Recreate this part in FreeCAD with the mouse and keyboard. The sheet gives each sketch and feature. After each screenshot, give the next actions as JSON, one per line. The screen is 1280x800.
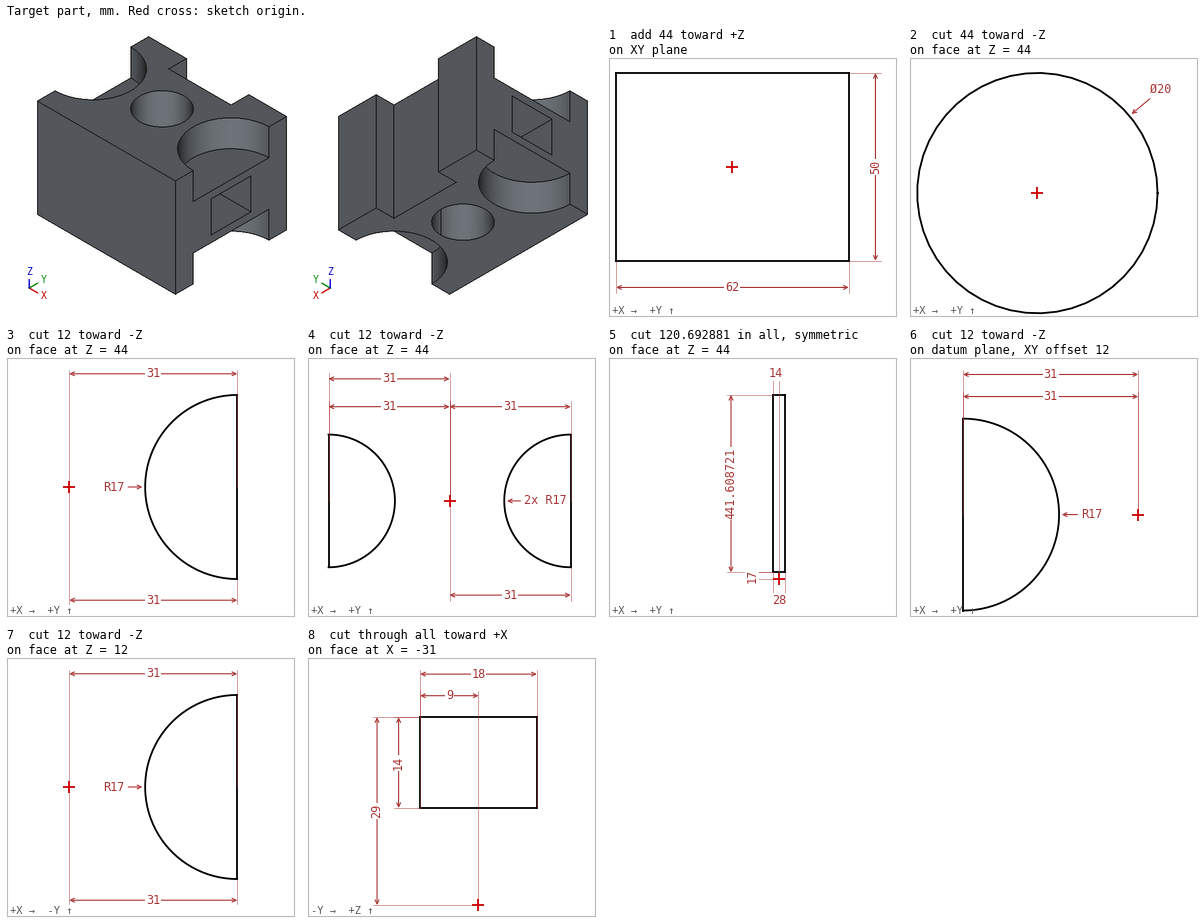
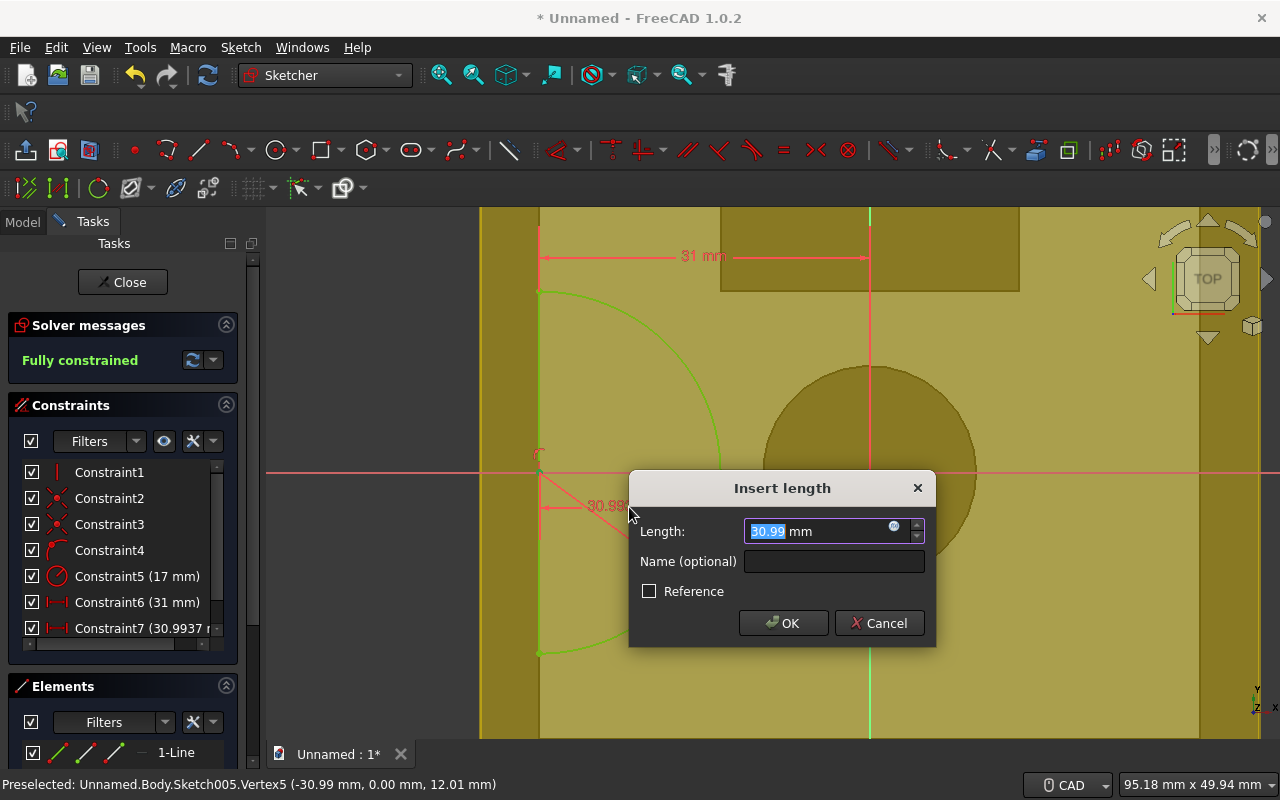
{"action": "type", "text": "31"}
{"action": "key", "text": "Return"}
{"action": "key", "text": "Escape"}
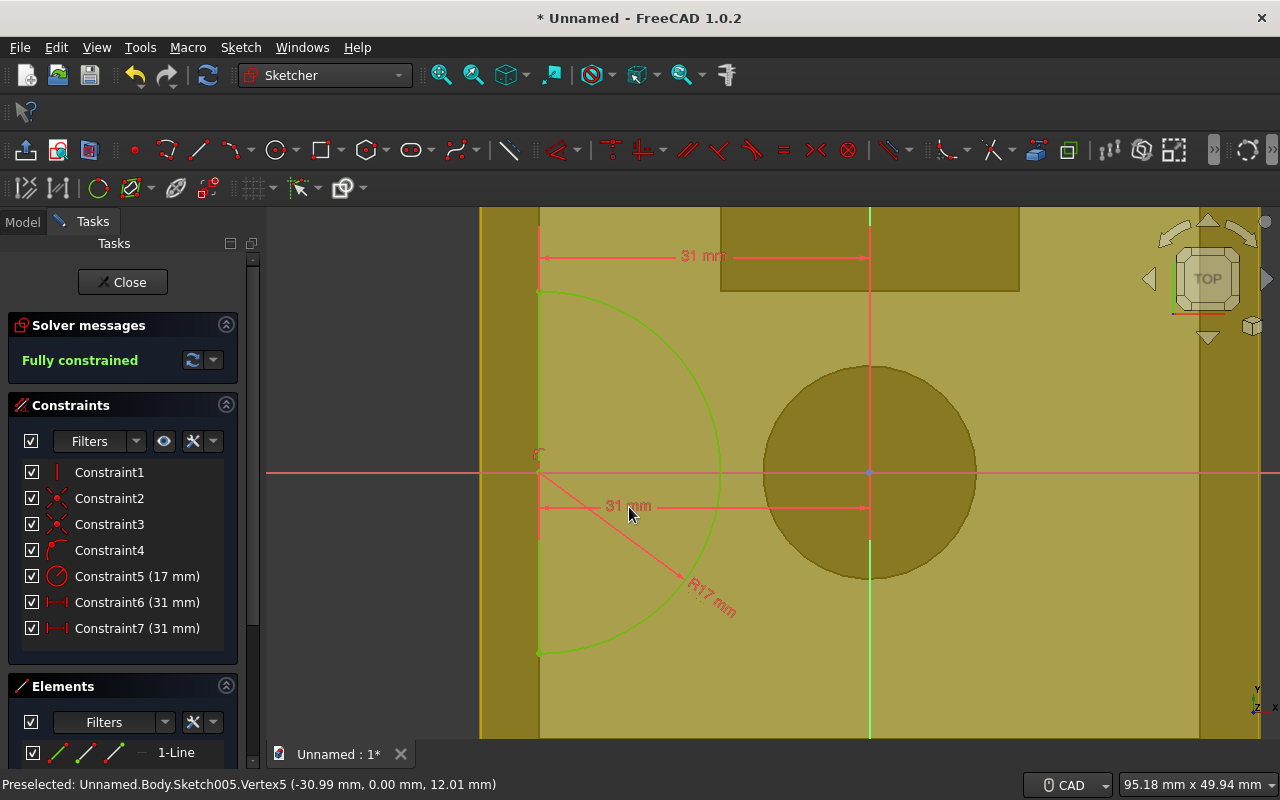
{"action": "left_click", "coordinate": [123, 282]}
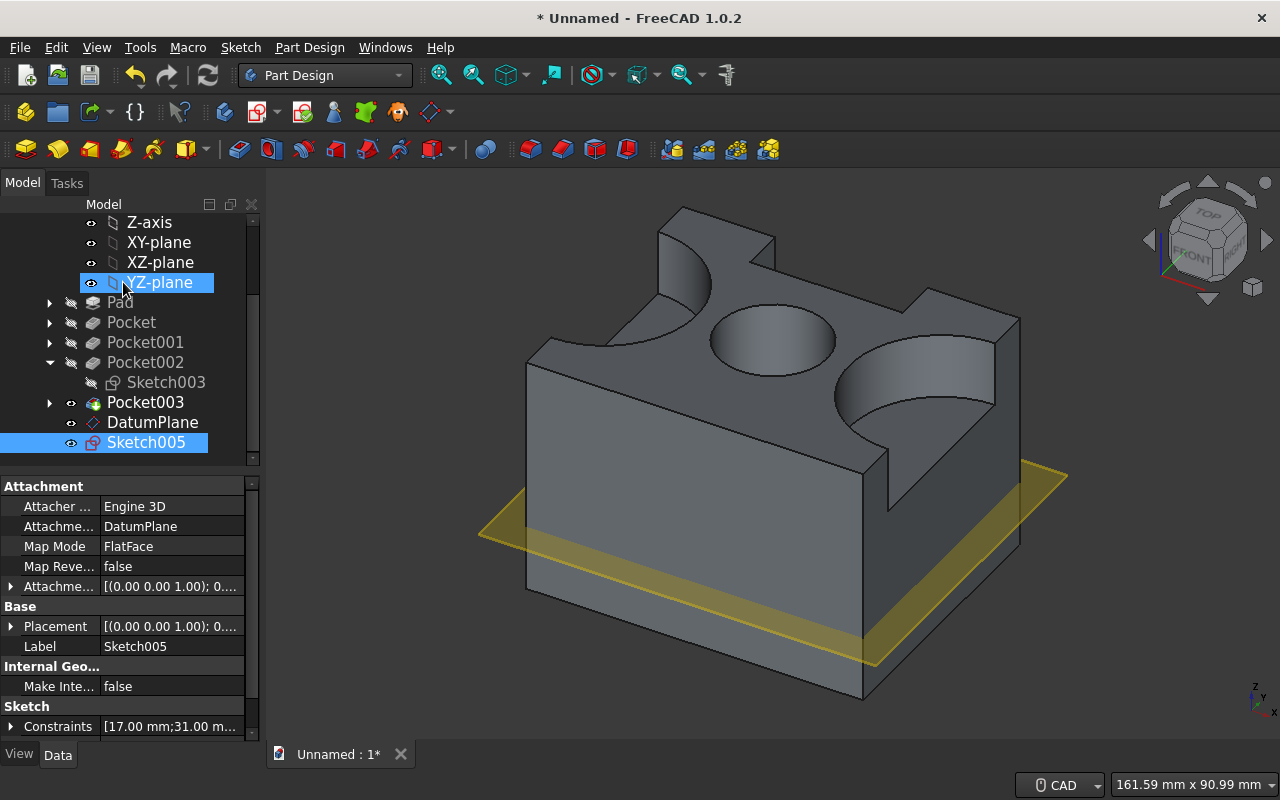
{"action": "left_click", "coordinate": [240, 150]}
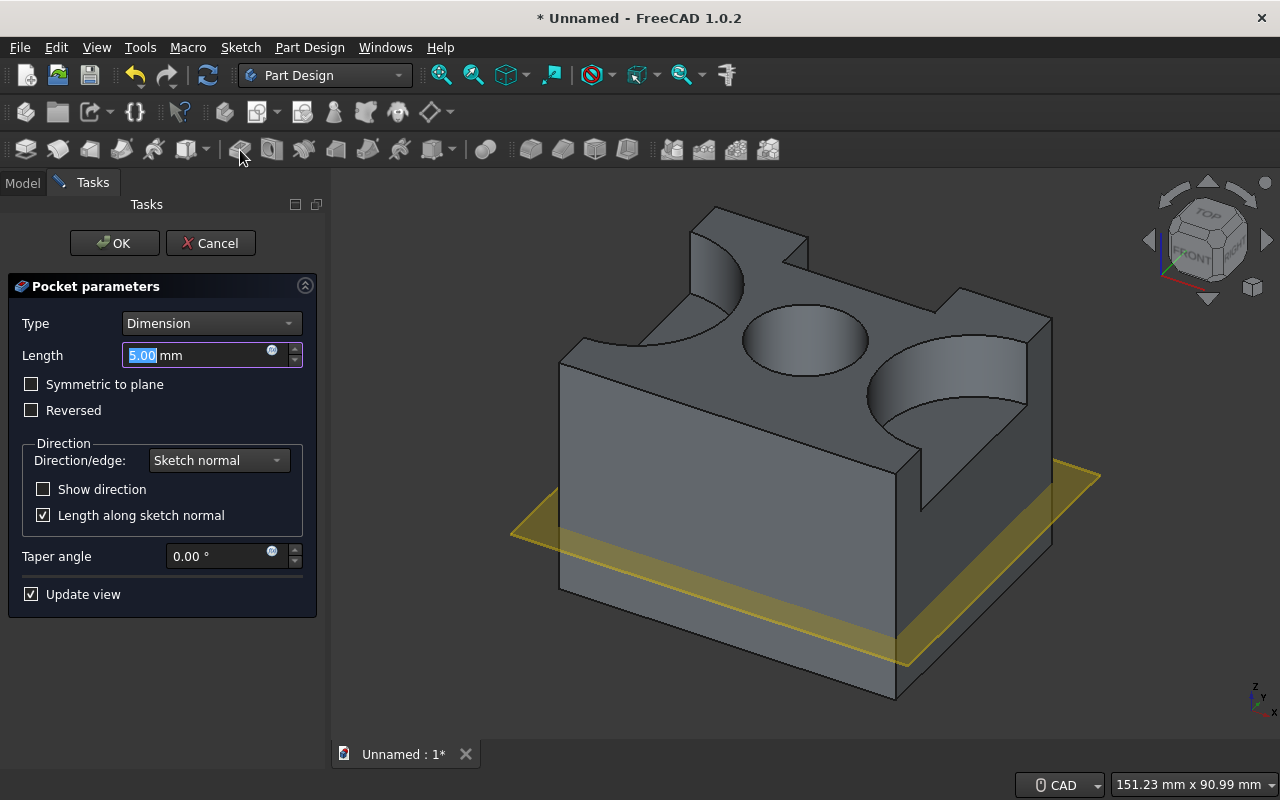
{"action": "type", "text": "12"}
{"action": "key", "text": "Tab"}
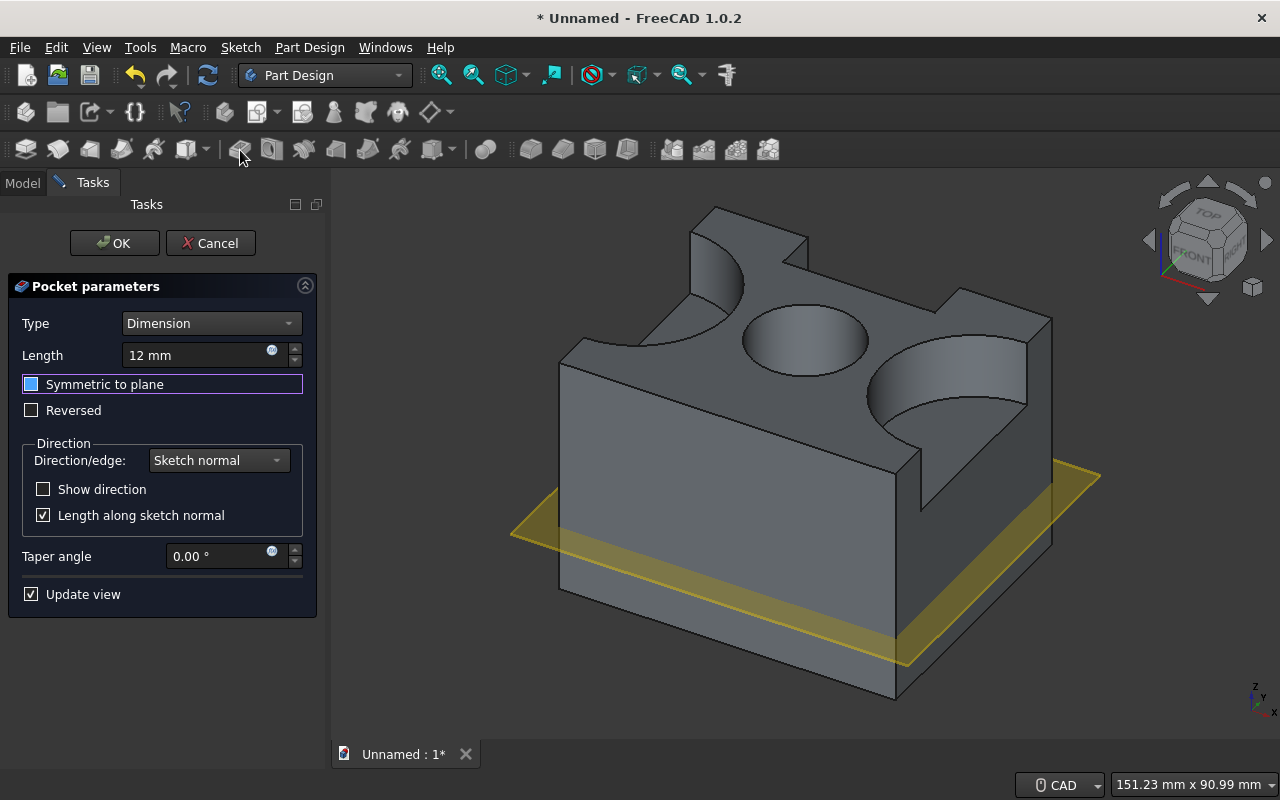
{"action": "left_click", "coordinate": [115, 243]}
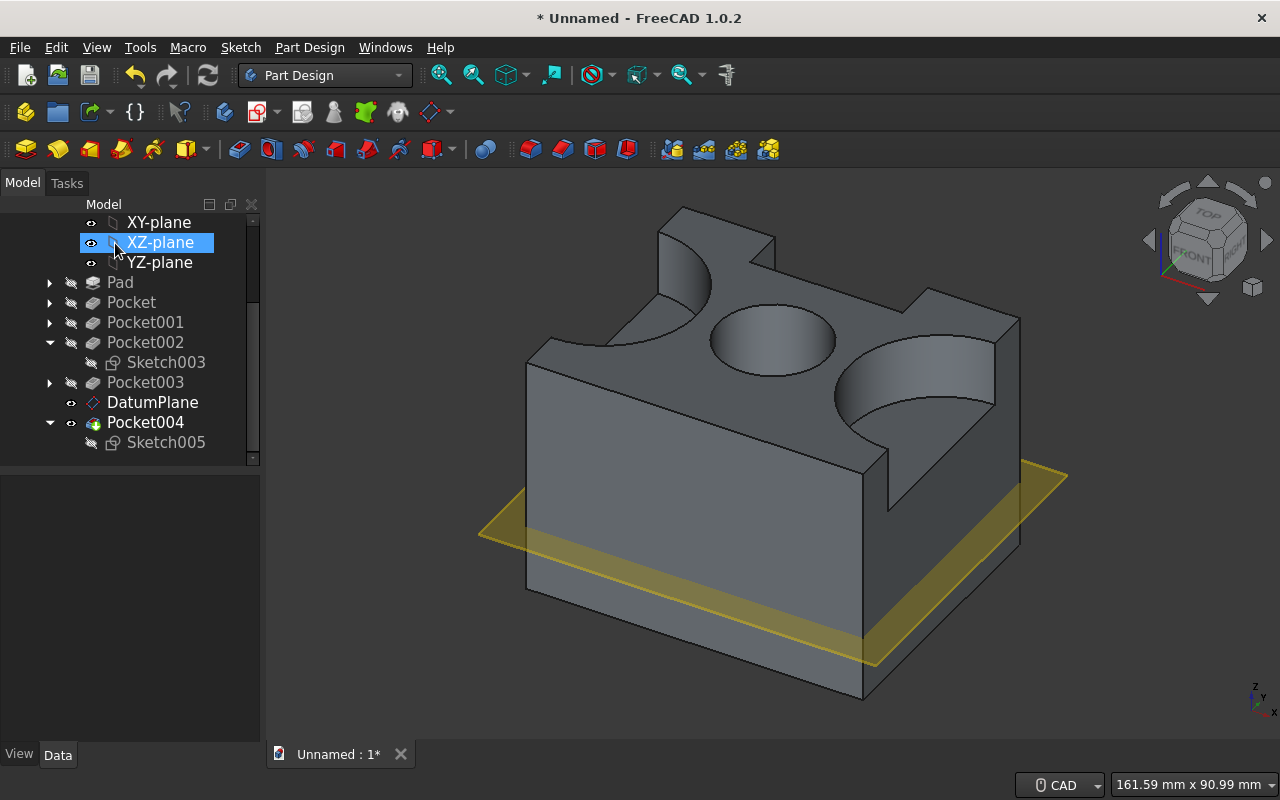
{"action": "left_click", "coordinate": [116, 403]}
{"action": "key", "text": "space"}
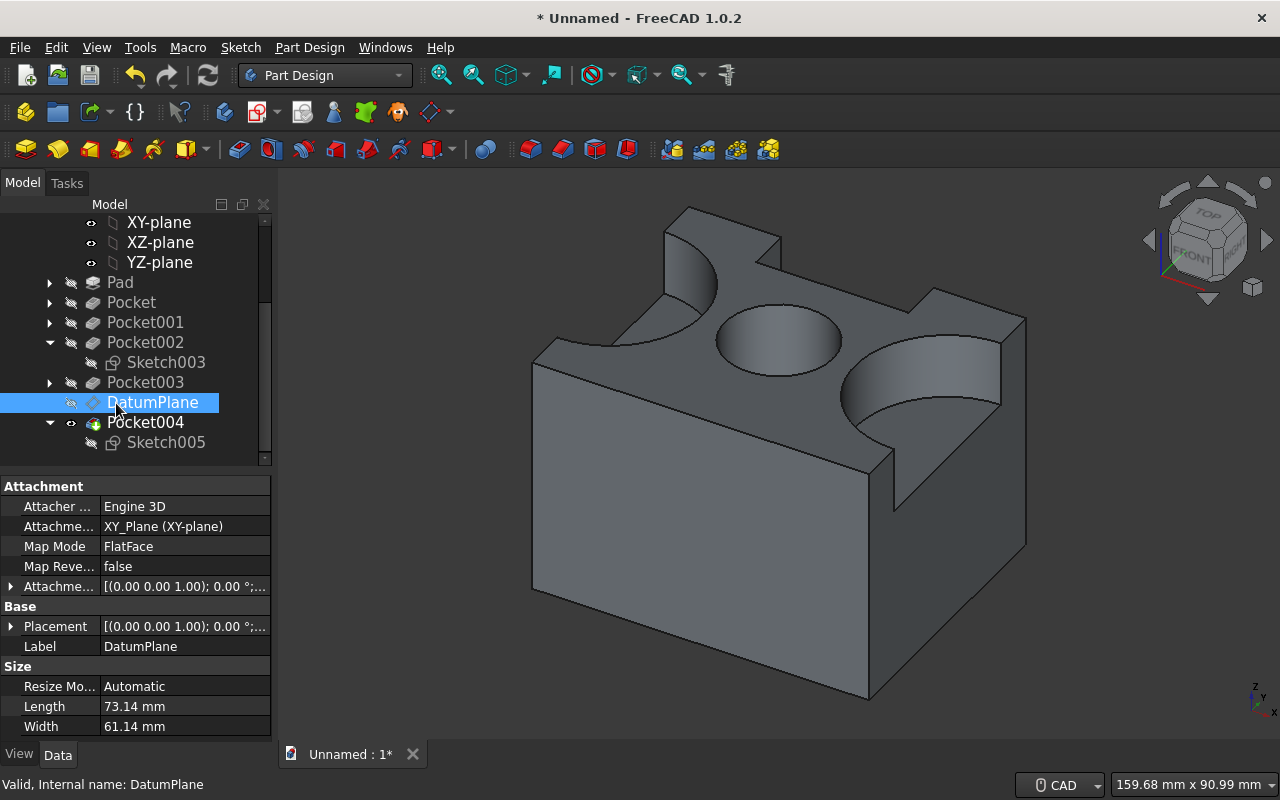
{"action": "key", "text": "5"}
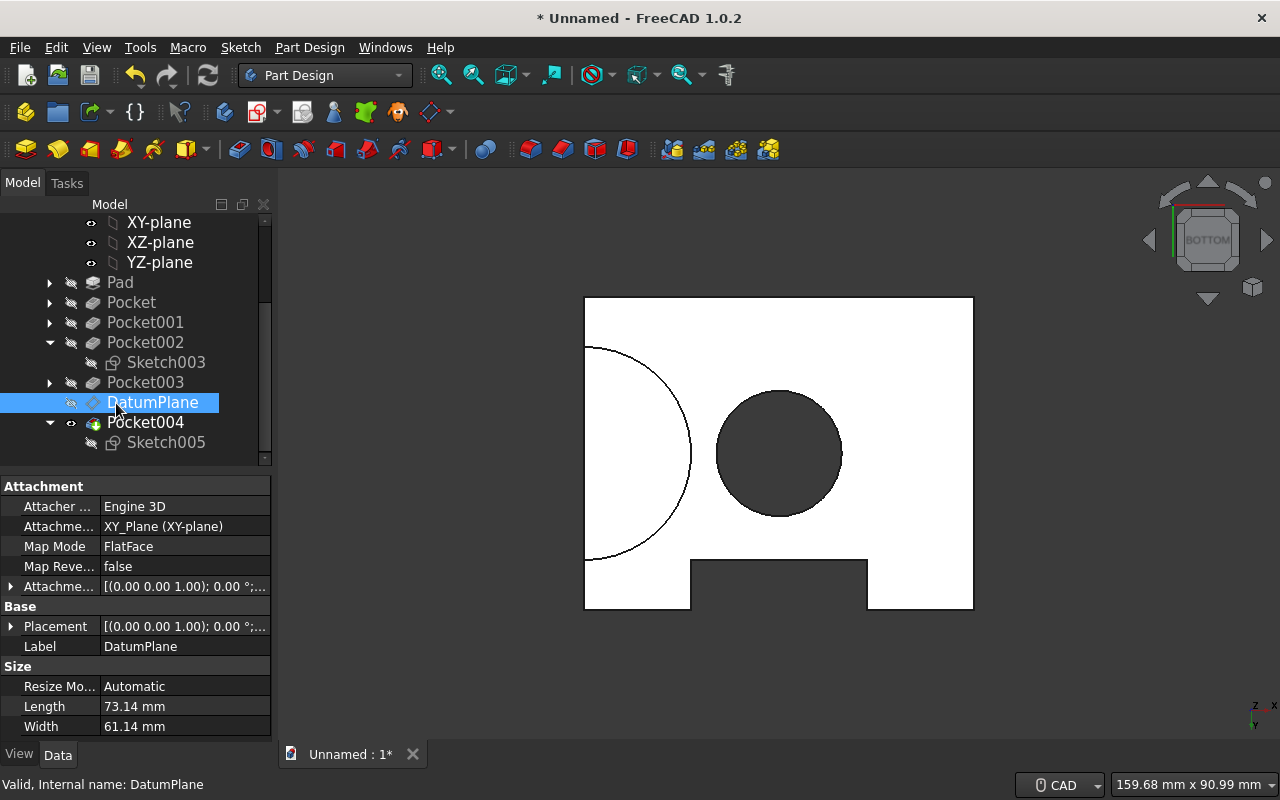
{"action": "left_click", "coordinate": [638, 452]}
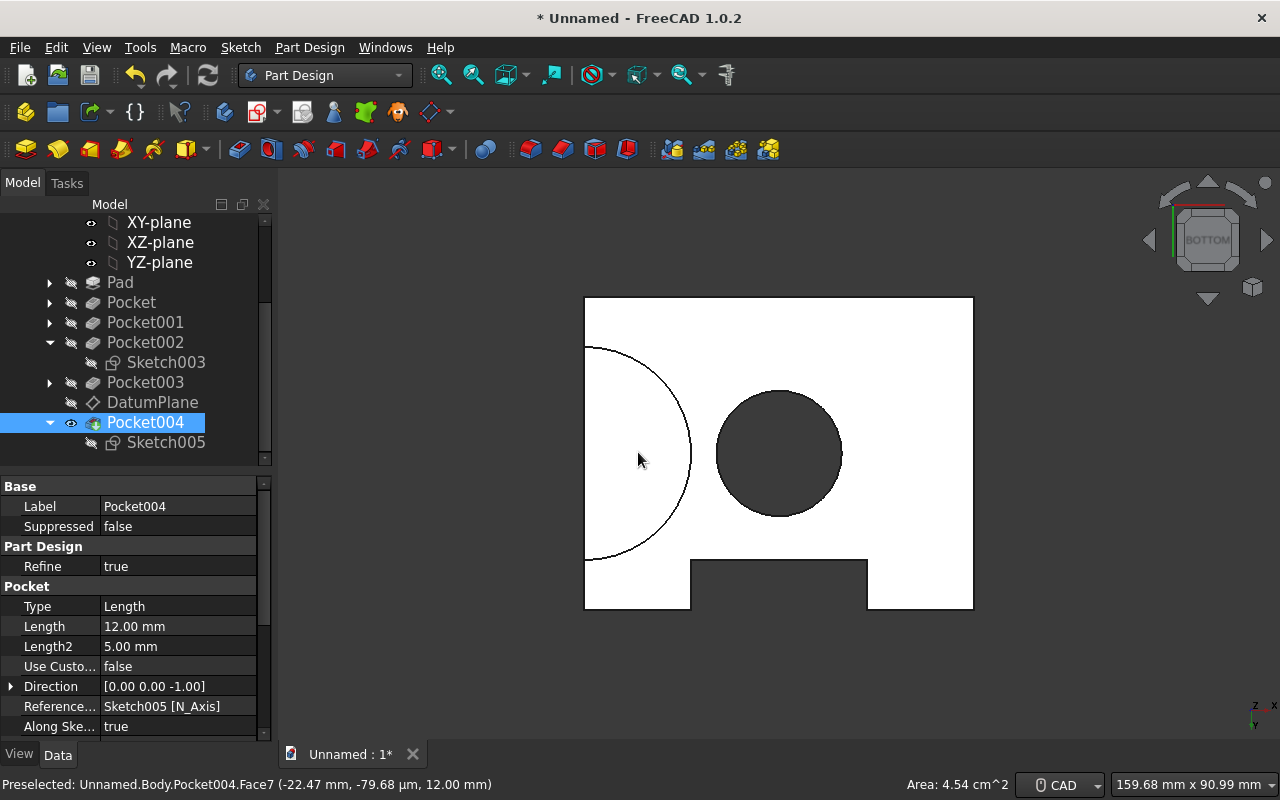
{"action": "left_click", "coordinate": [258, 112]}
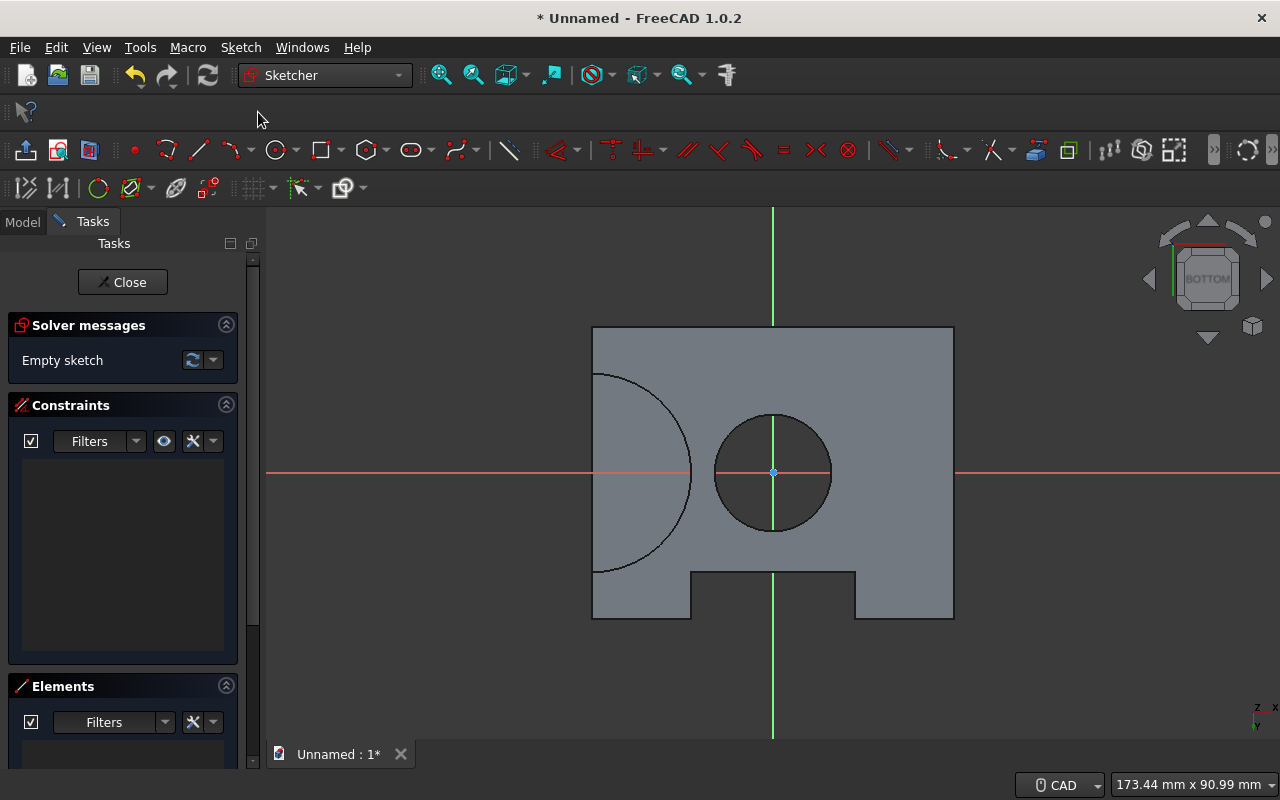
{"action": "scroll", "coordinate": [1057, 473], "scroll_direction": "up", "scroll_amount": 3}